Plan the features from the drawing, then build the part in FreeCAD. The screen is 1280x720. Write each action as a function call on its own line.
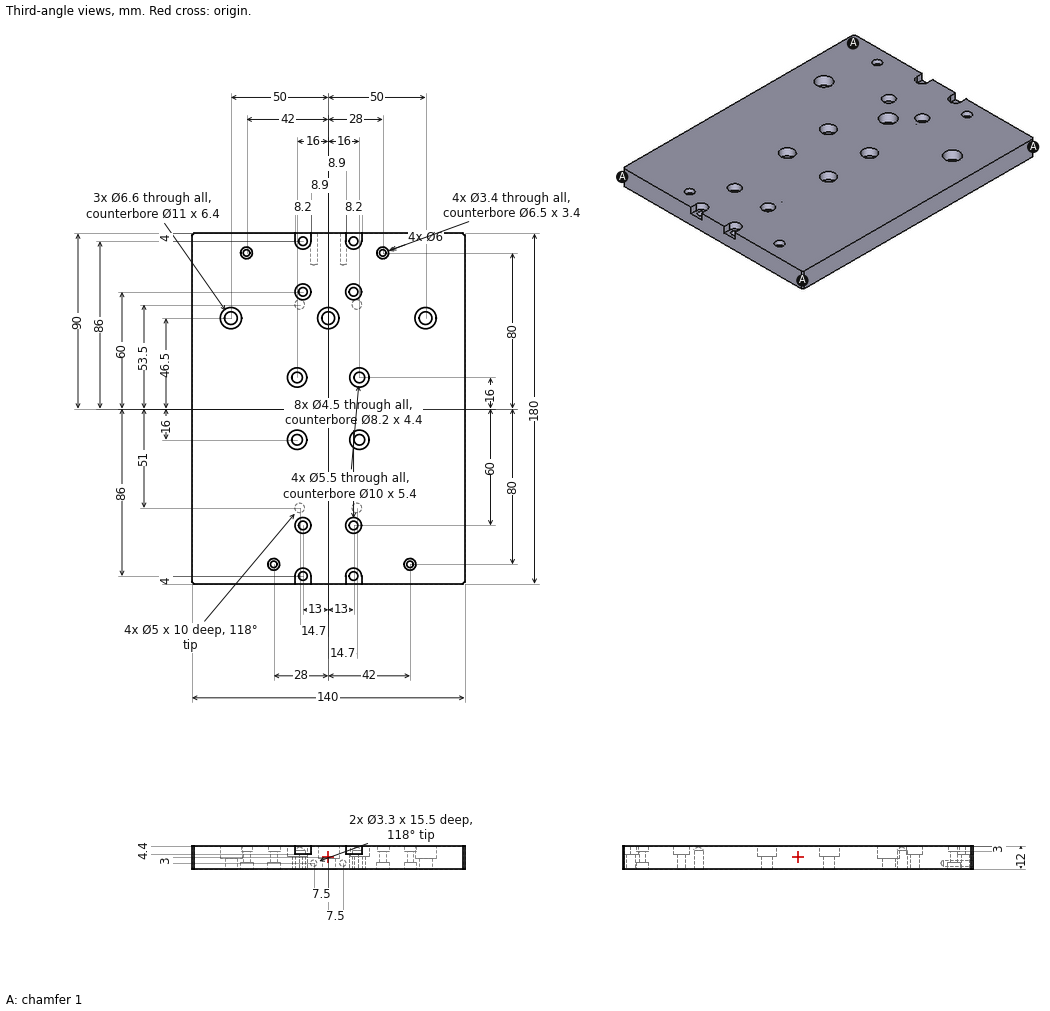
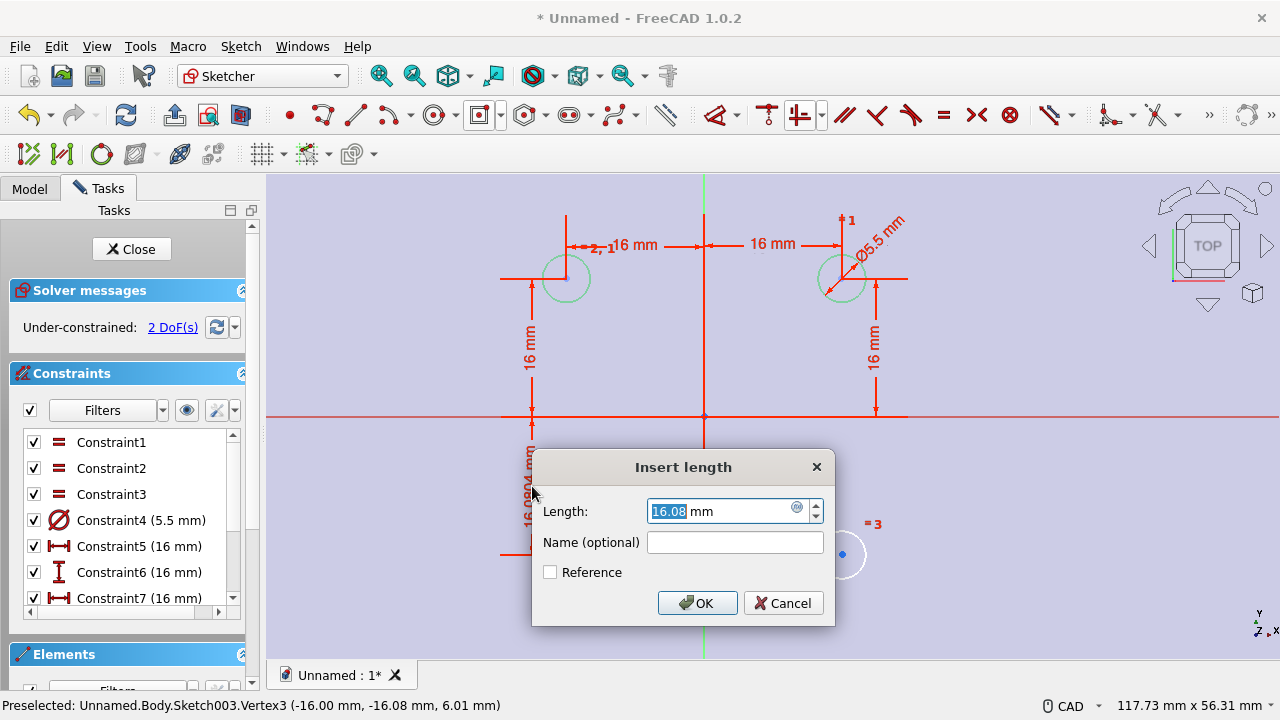
text(16)
key(Return)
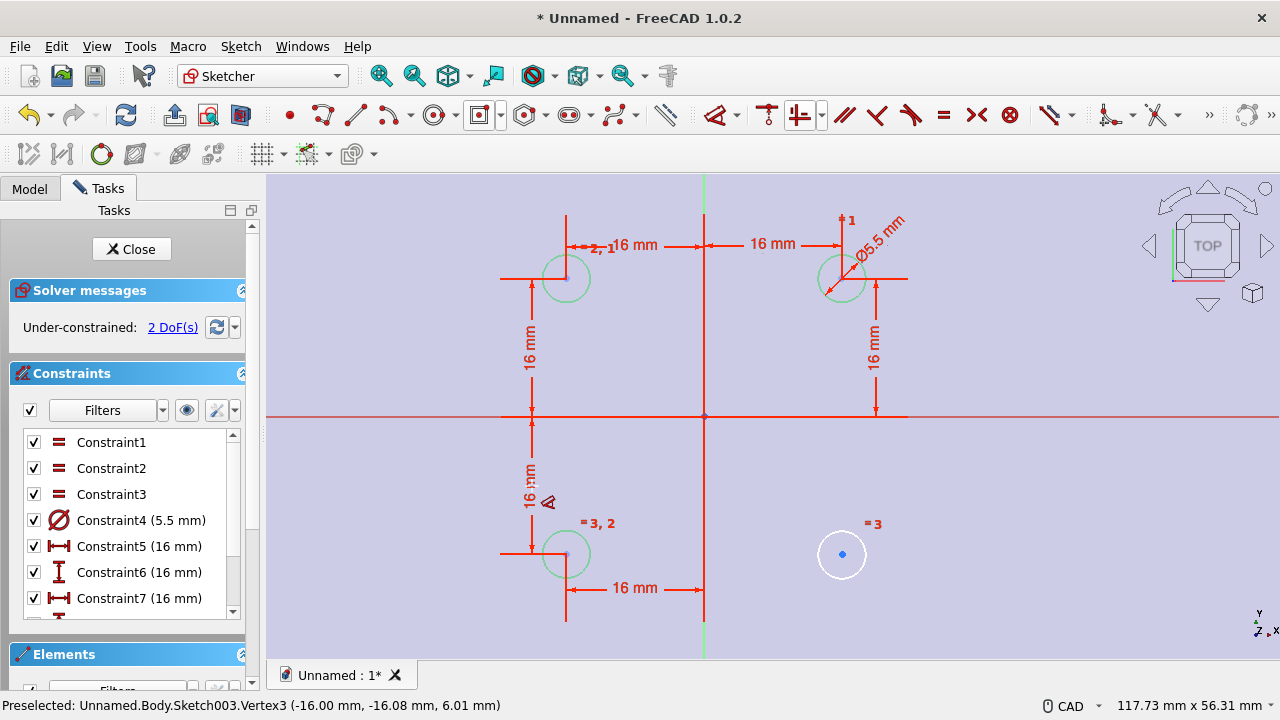
click(842, 555)
click(773, 589)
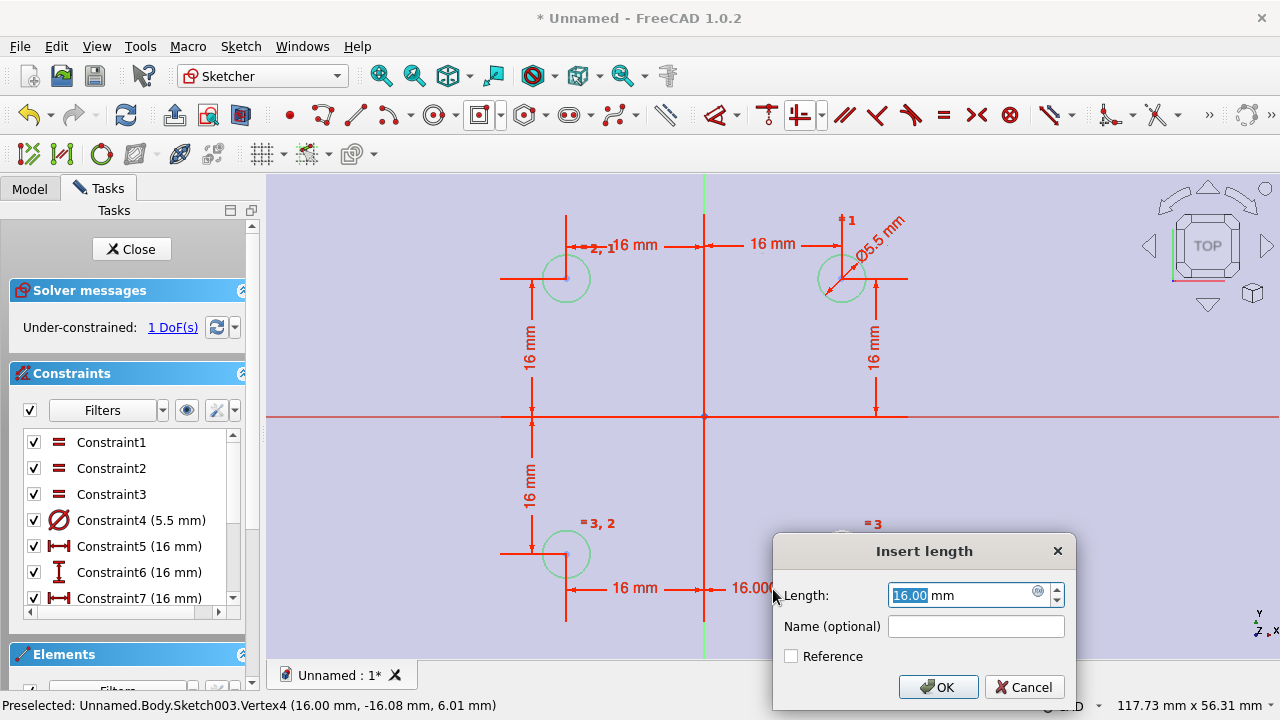
text(16)
key(Return)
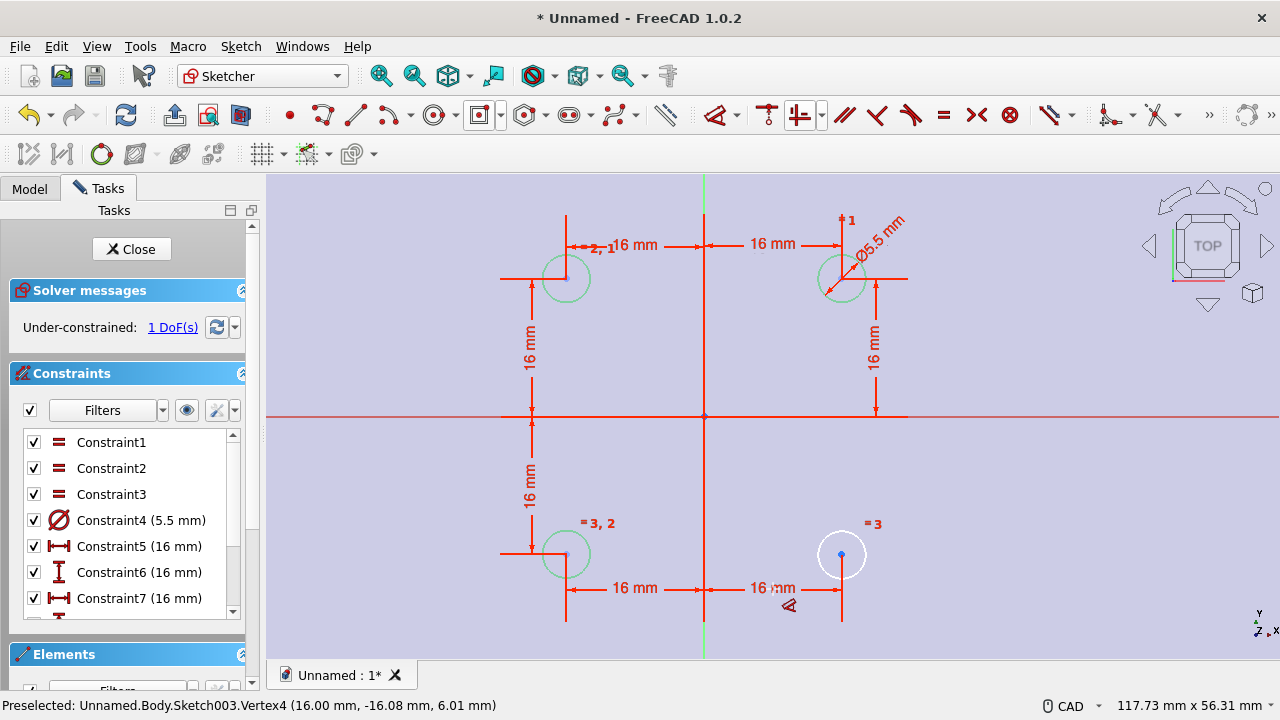
click(842, 555)
click(876, 486)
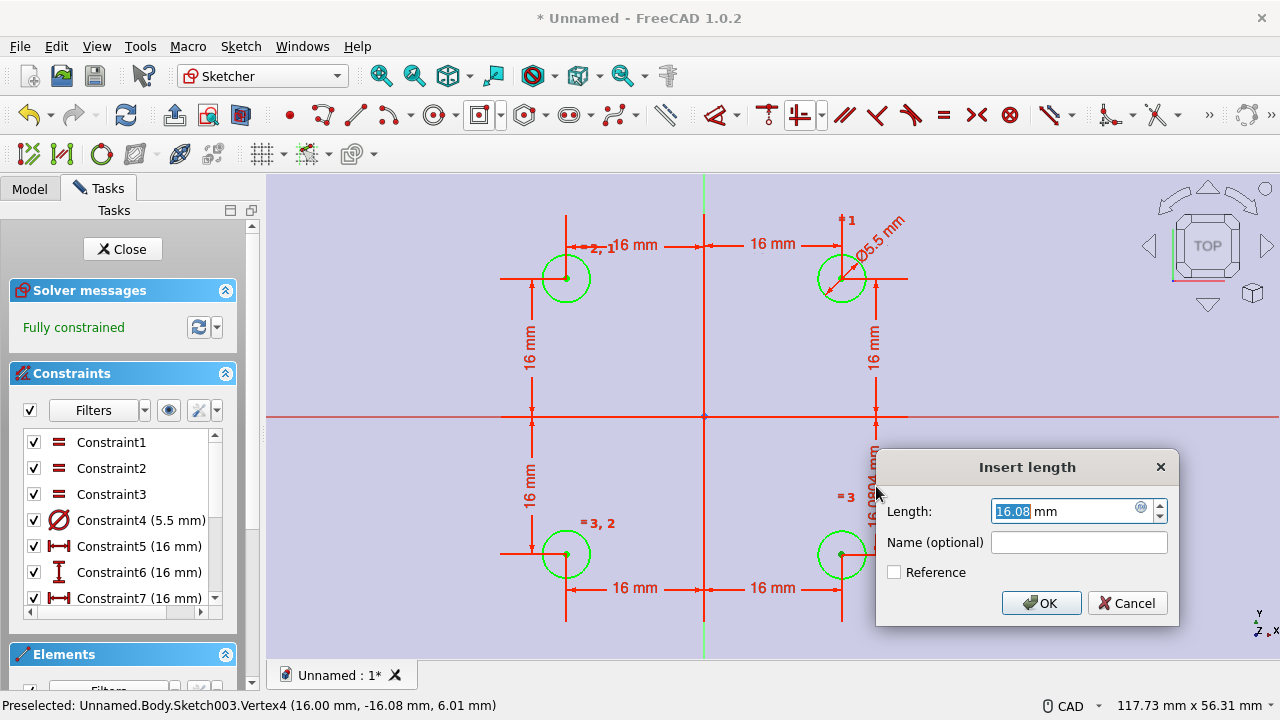
text(16)
key(Return)
key(Escape)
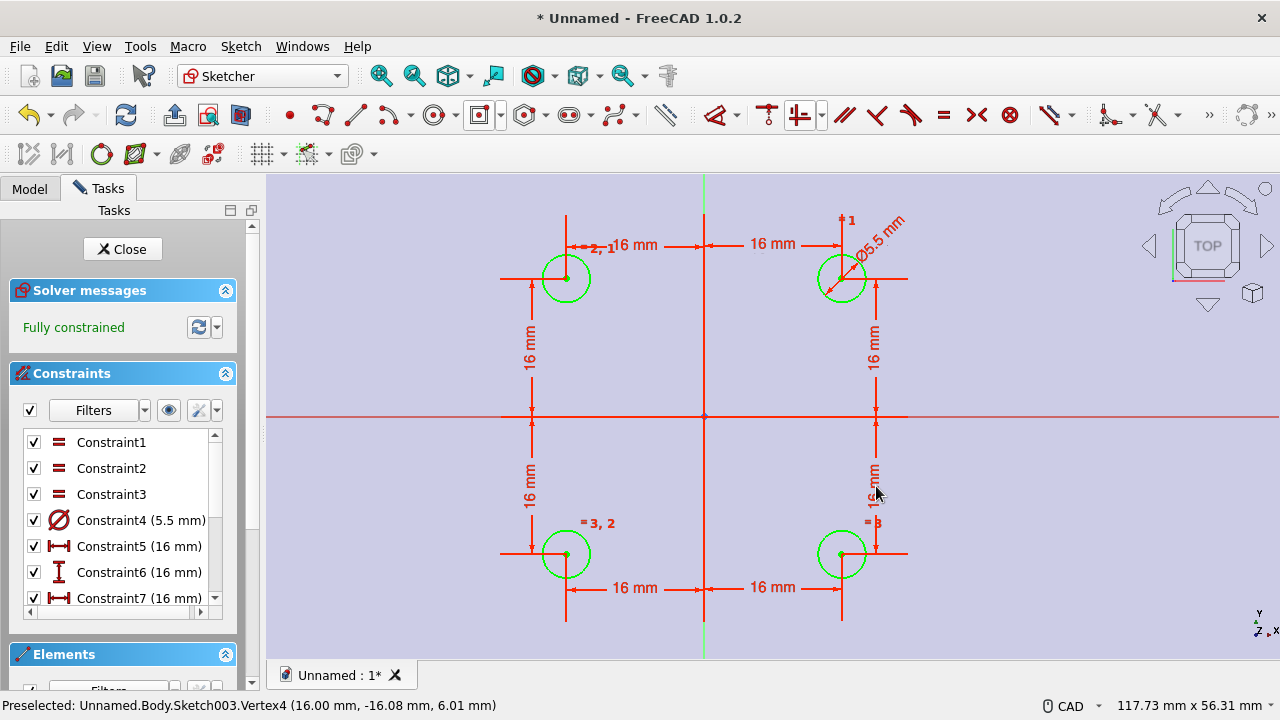
click(123, 249)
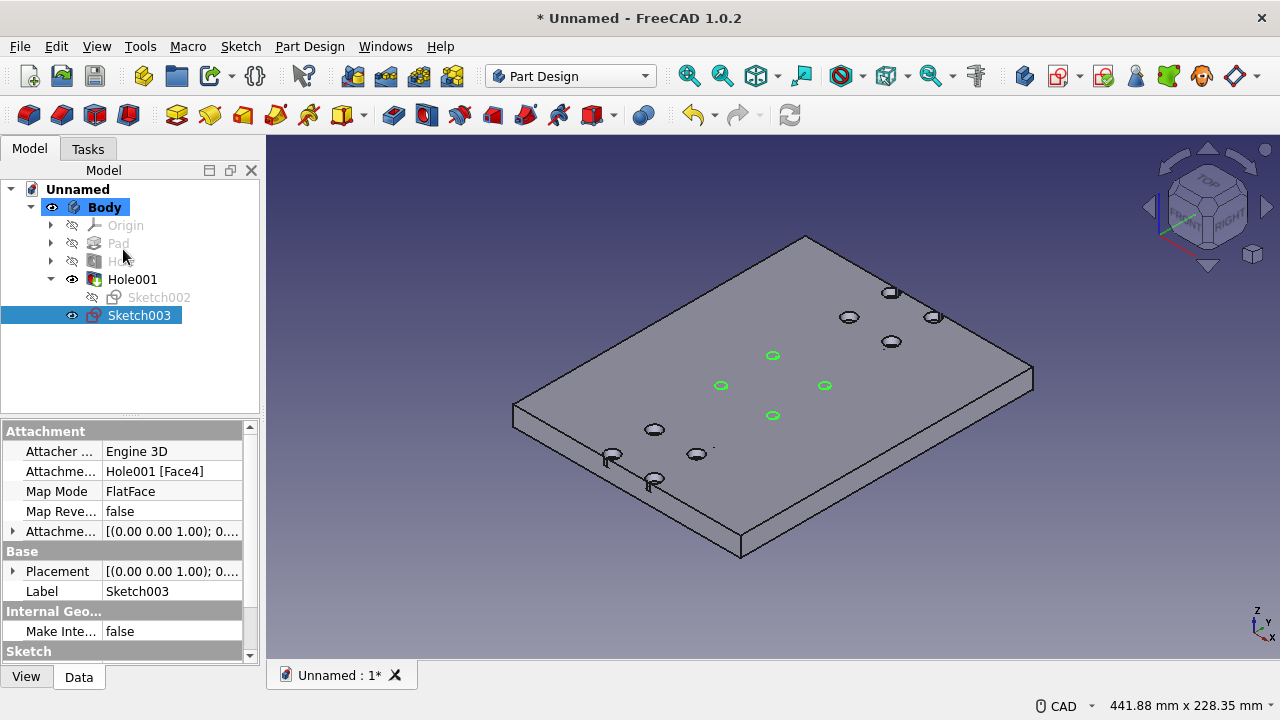
click(427, 116)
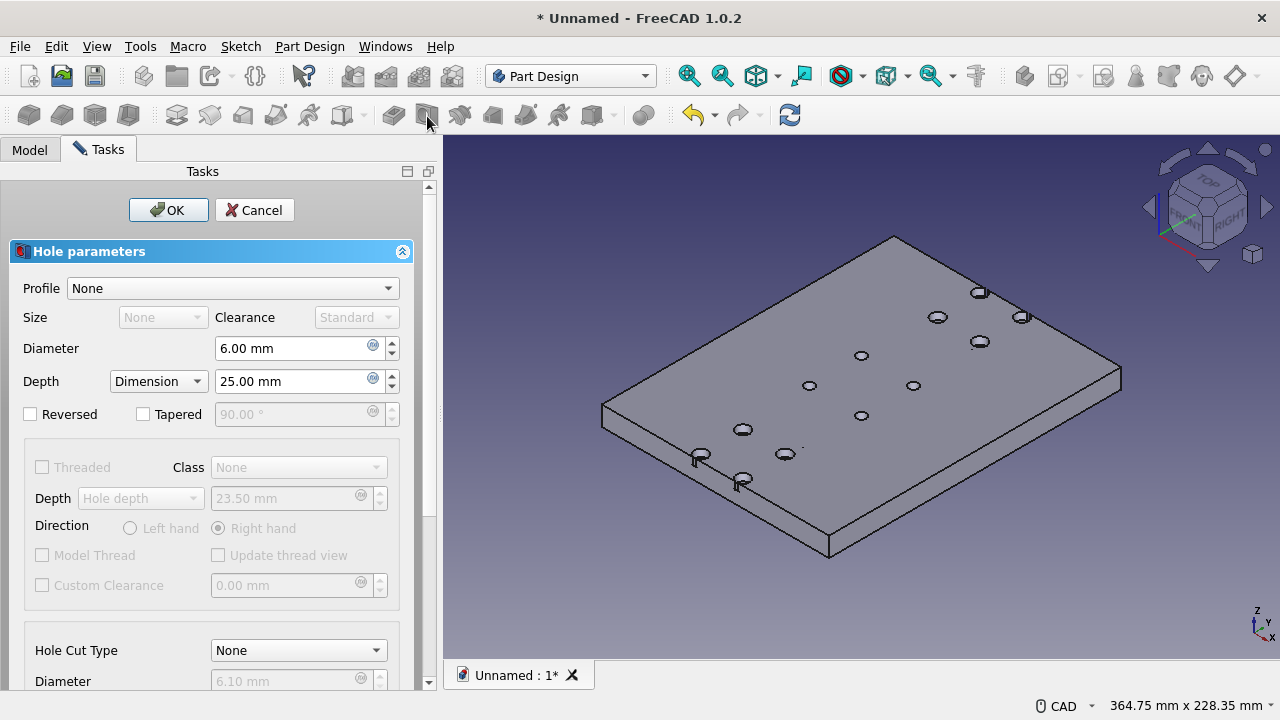
triple_click(300, 348)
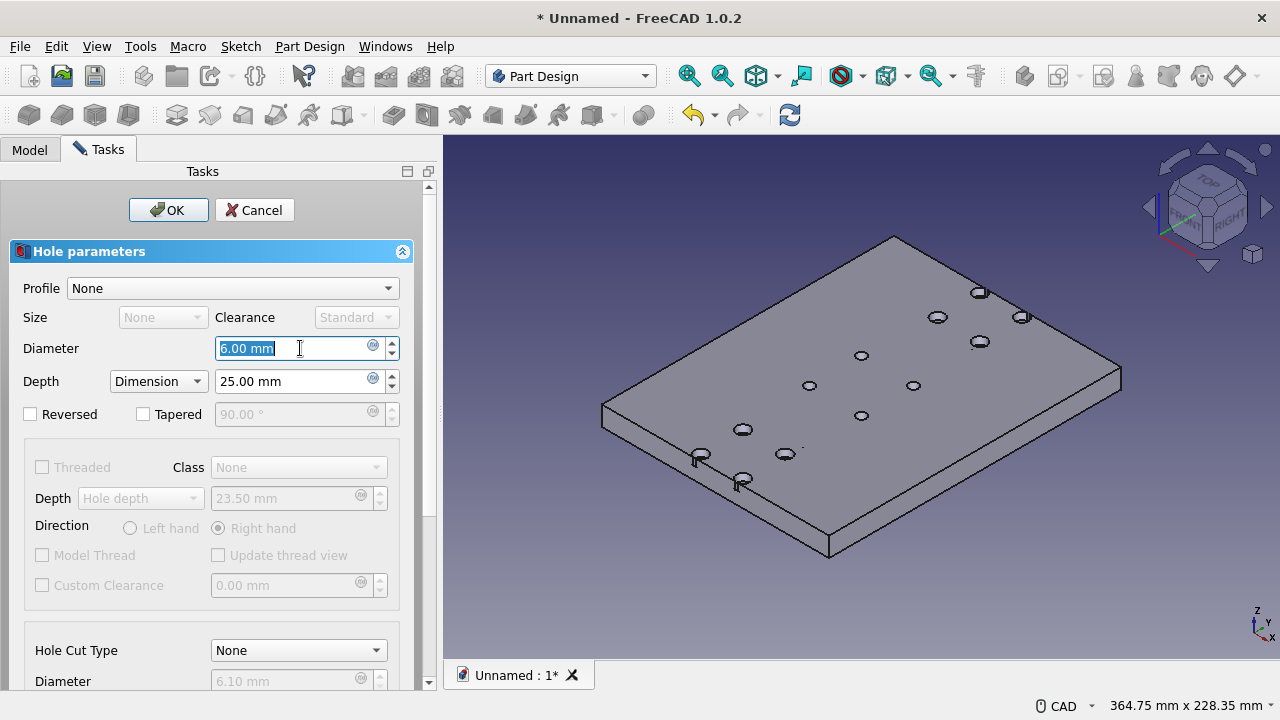
text(5.5)
key(Tab)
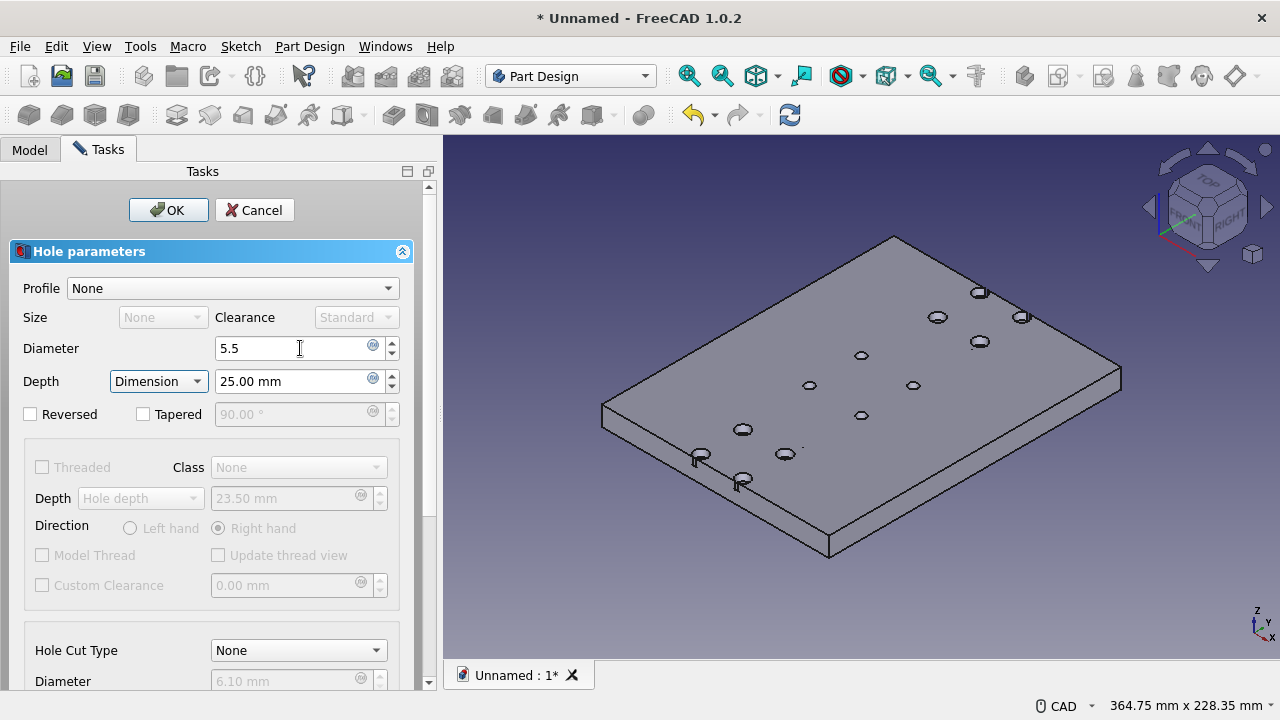
click(160, 382)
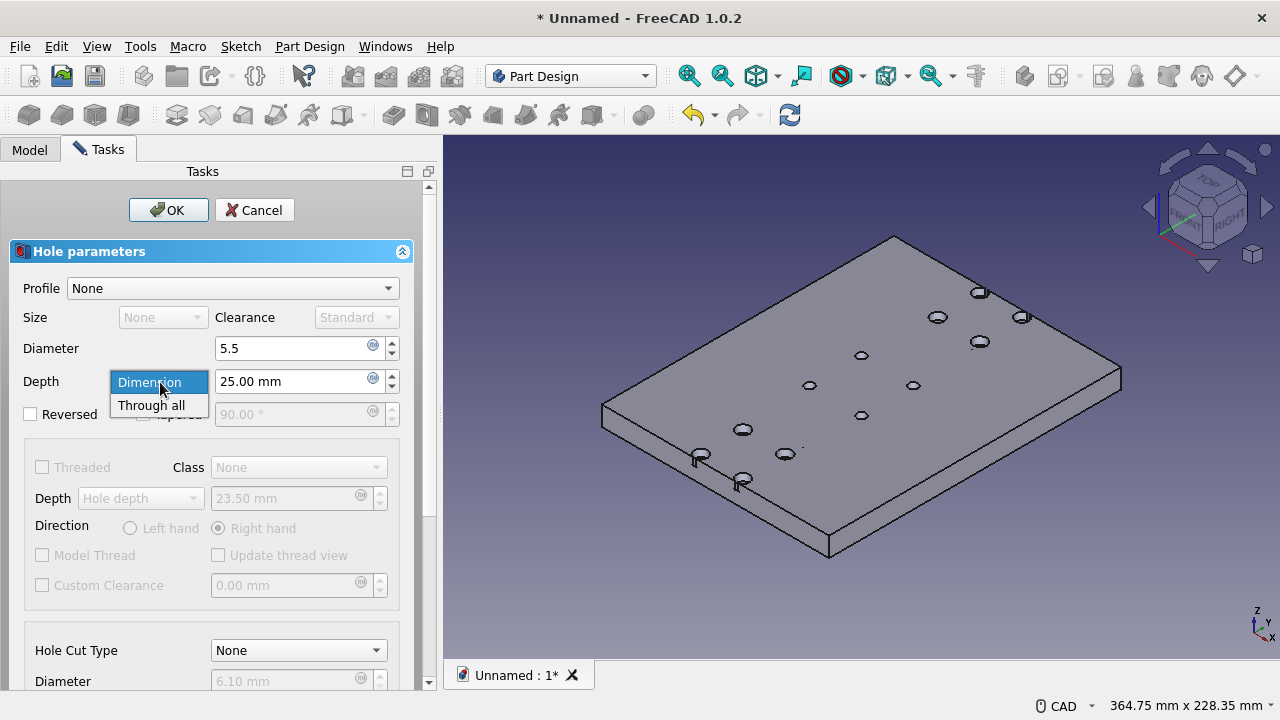
click(158, 406)